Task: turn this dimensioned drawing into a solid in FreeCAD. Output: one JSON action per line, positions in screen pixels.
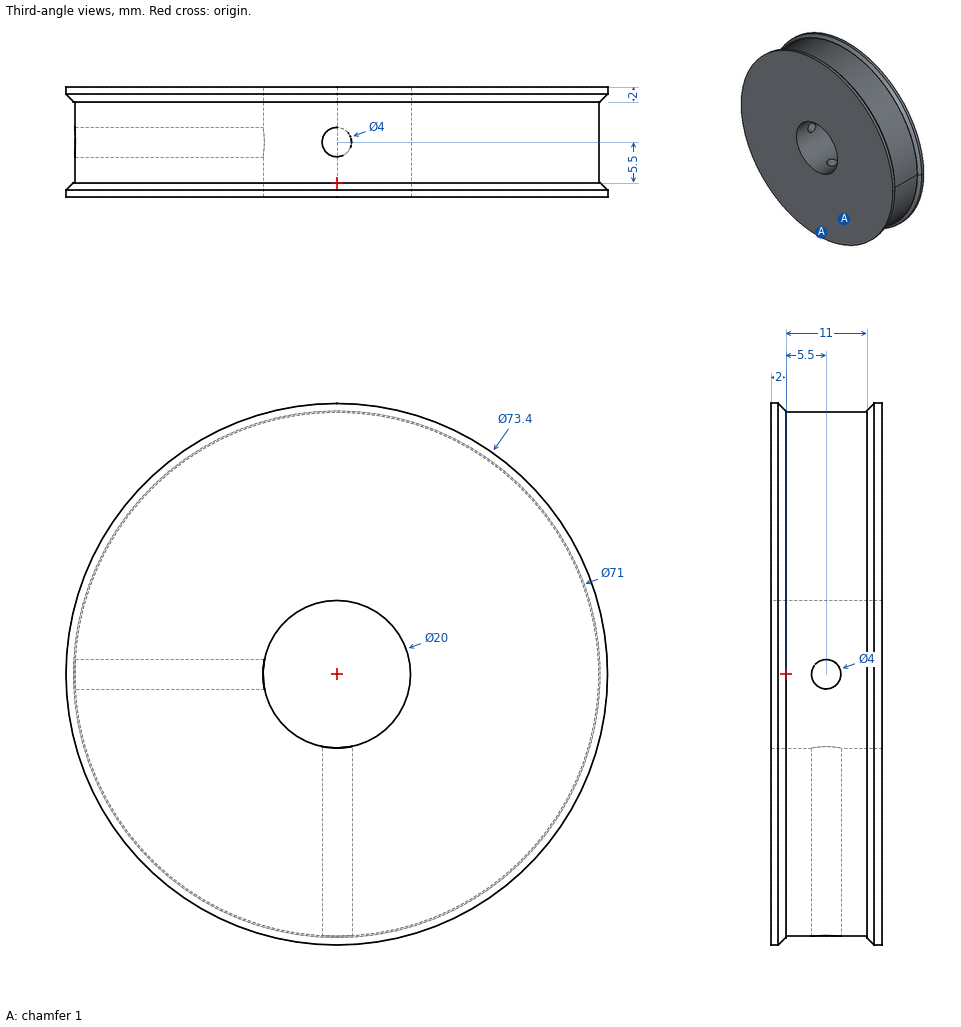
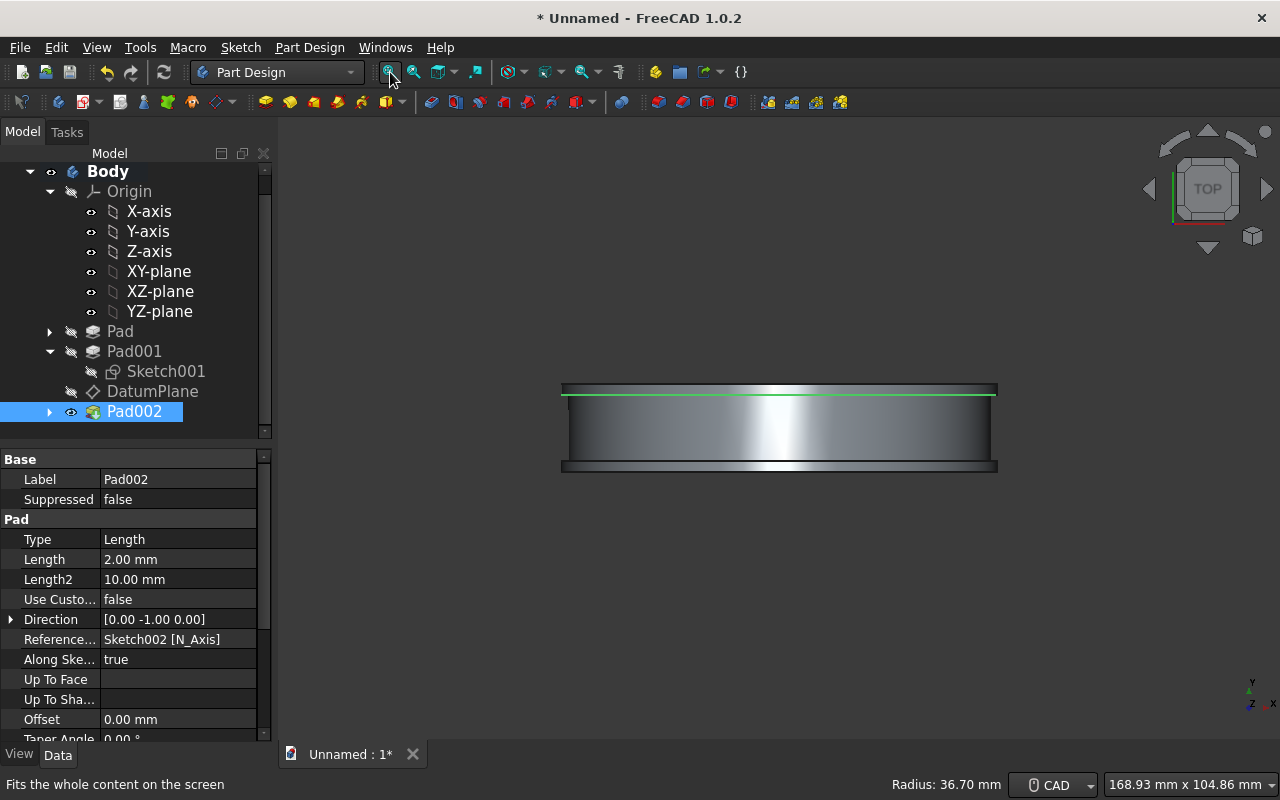
{"action": "left_click", "coordinate": [603, 460], "text": "ctrl"}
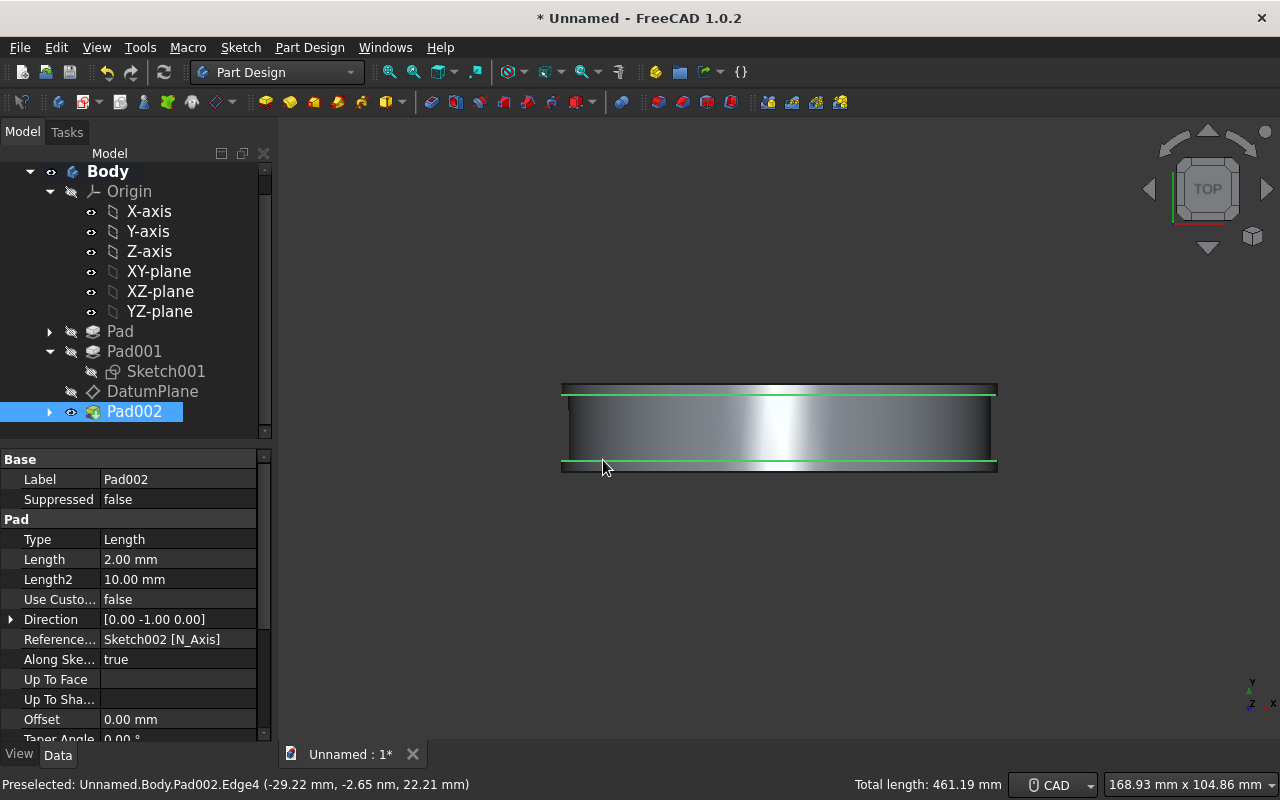
{"action": "left_click", "coordinate": [684, 102]}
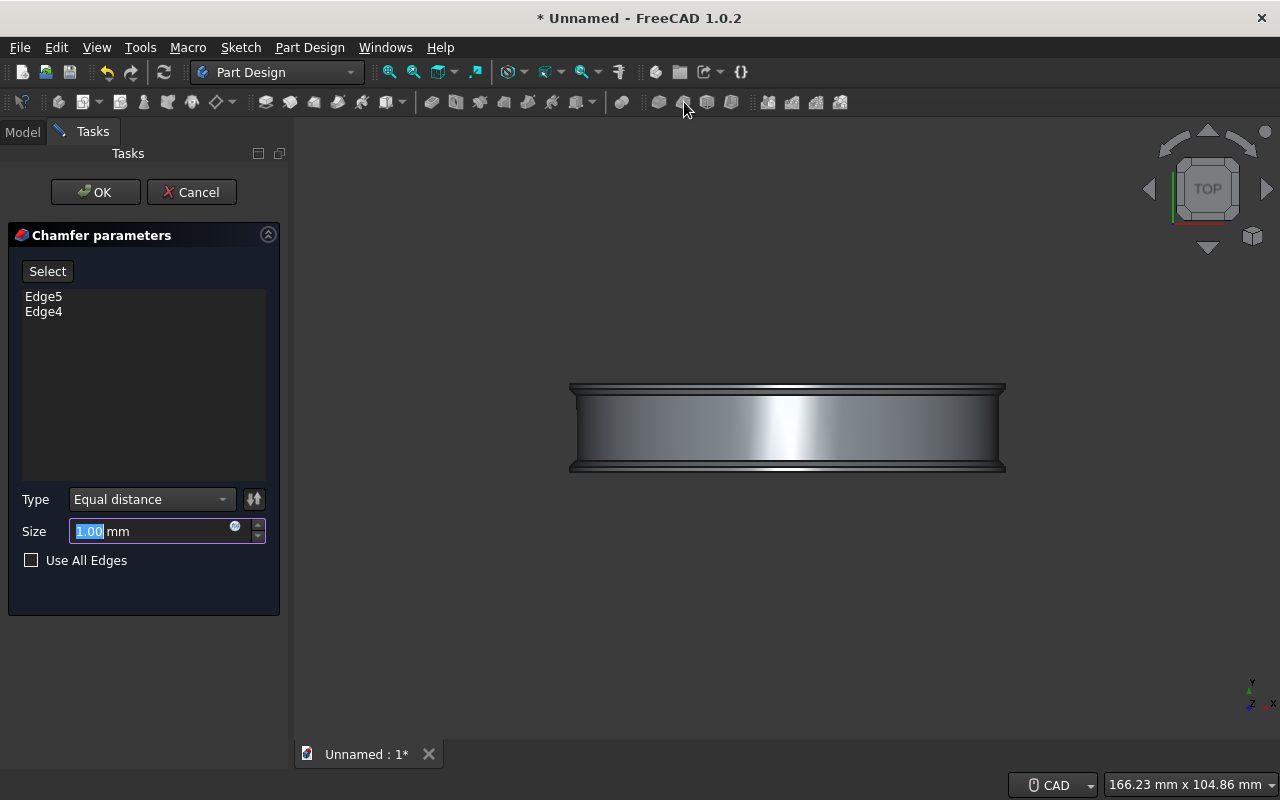
{"action": "type", "text": "1"}
{"action": "key", "text": "Tab"}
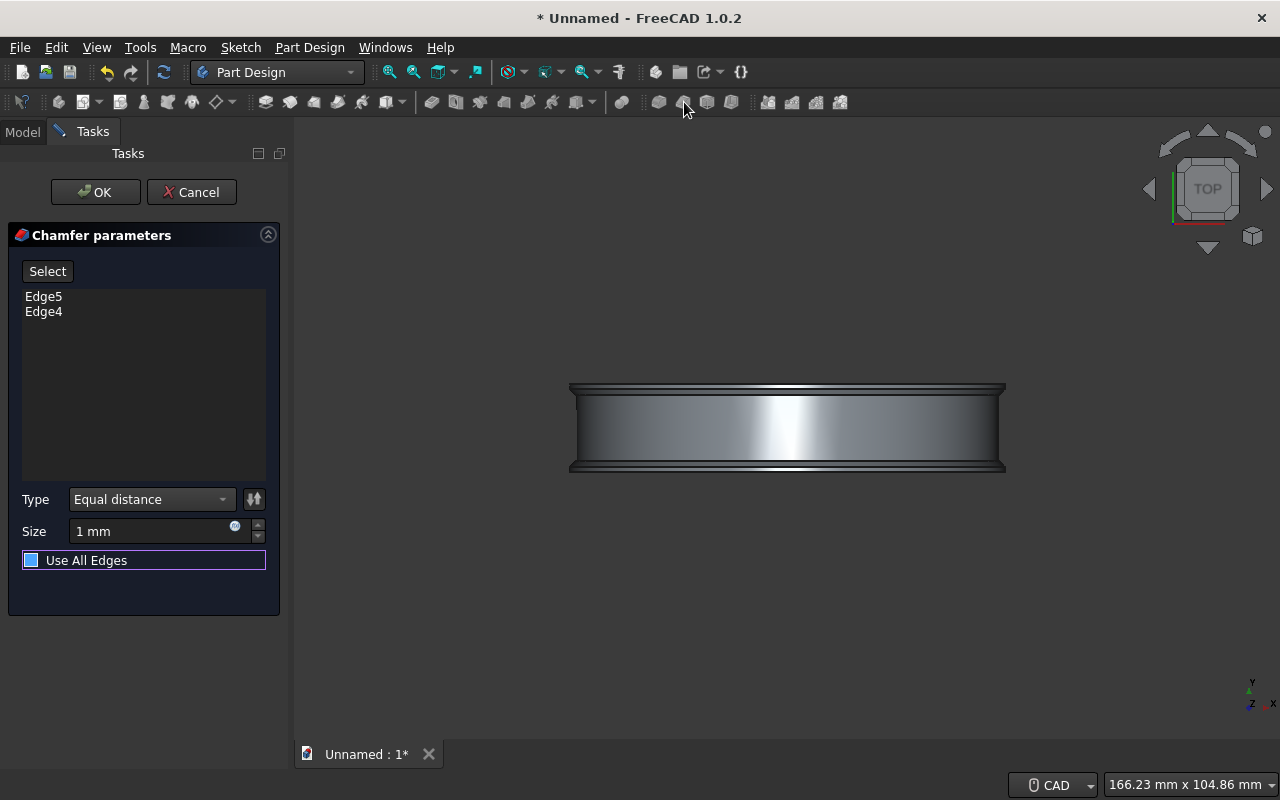
{"action": "left_click", "coordinate": [96, 192]}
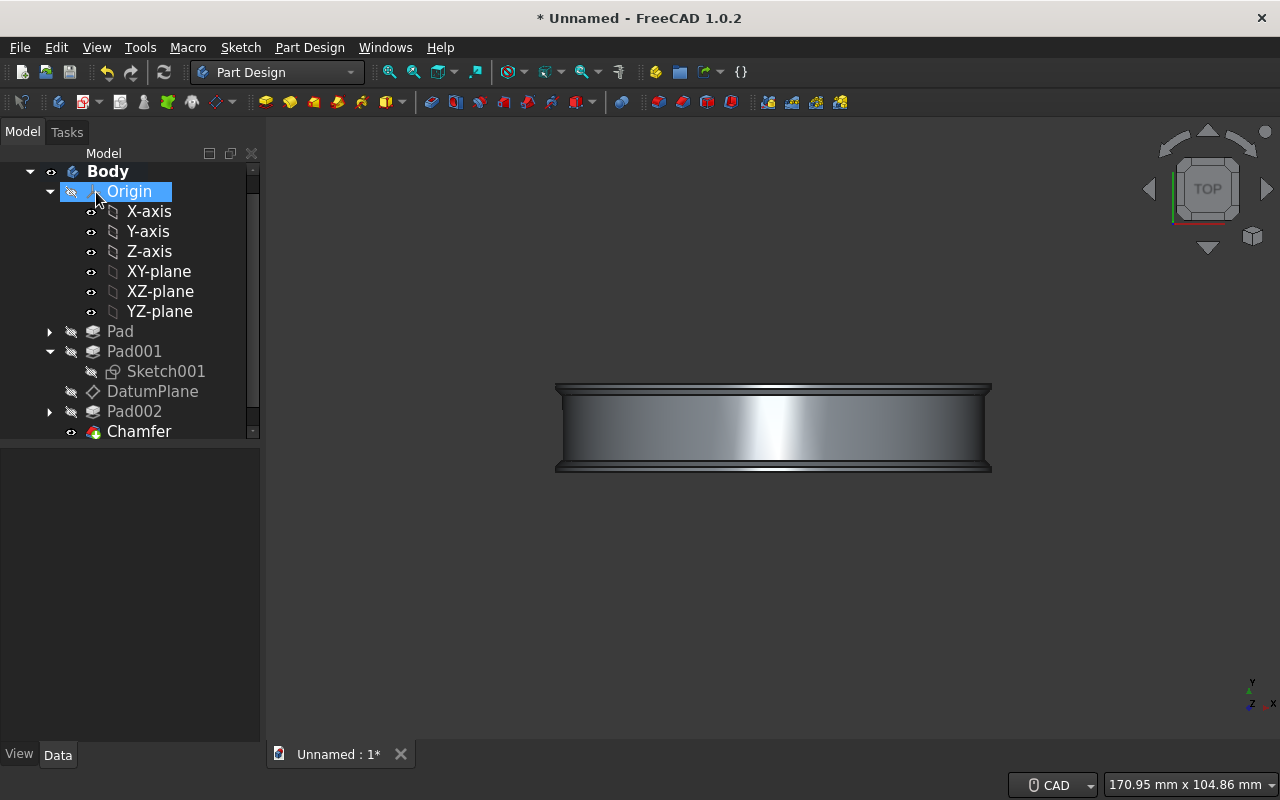
{"action": "left_click", "coordinate": [390, 72]}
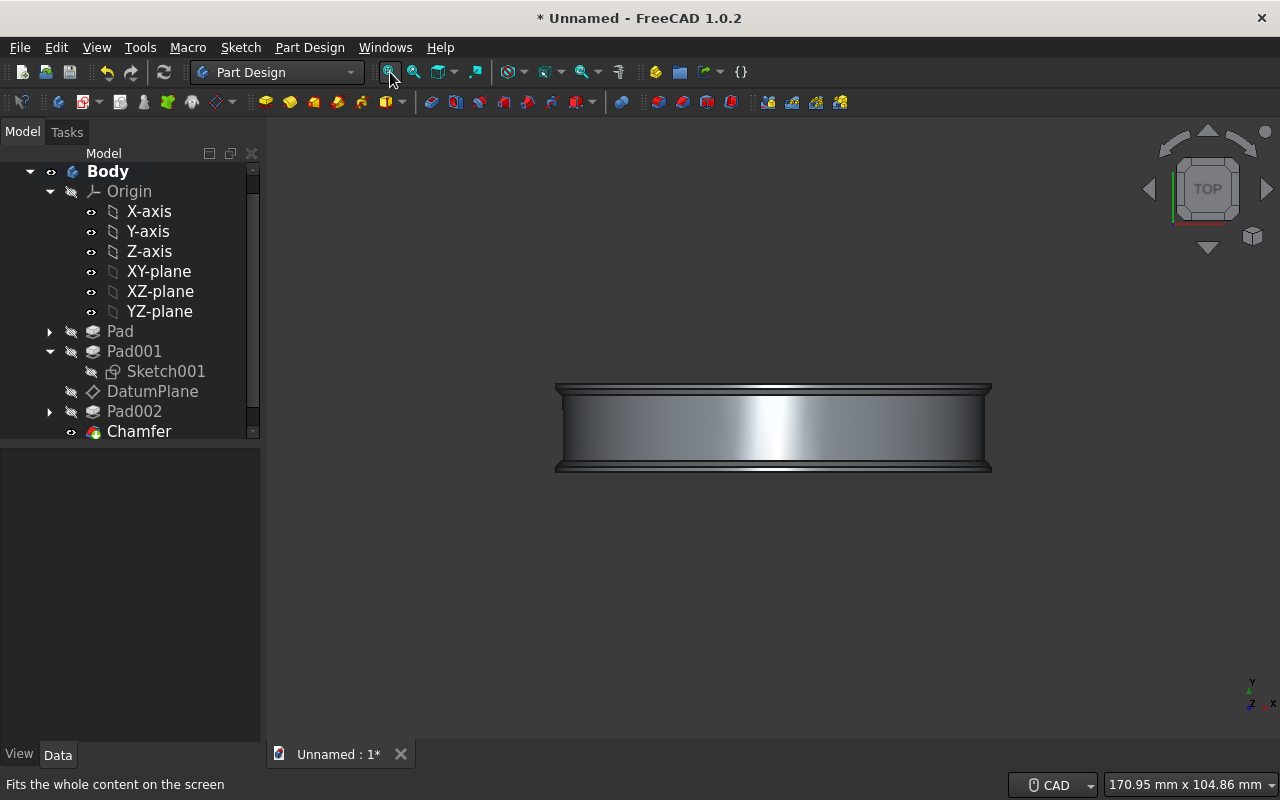
{"action": "left_click", "coordinate": [84, 102]}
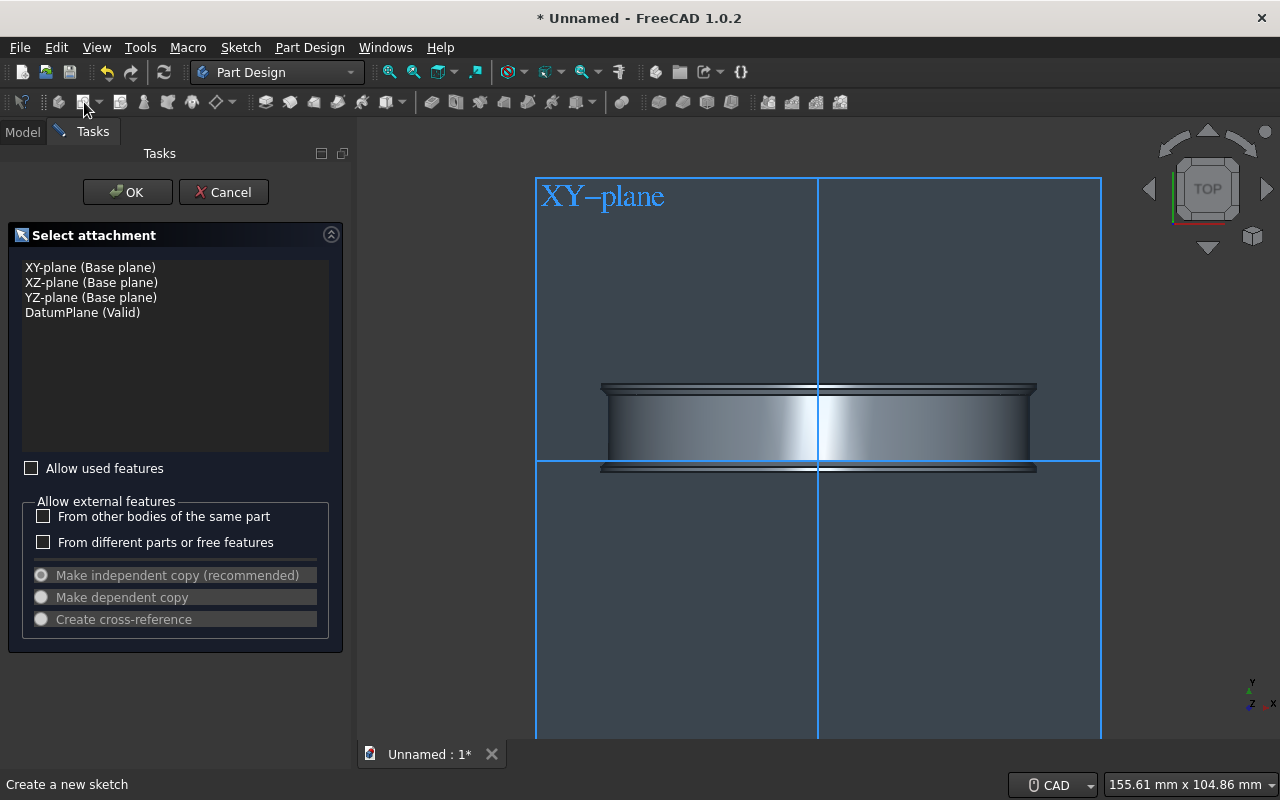
{"action": "left_click", "coordinate": [82, 268]}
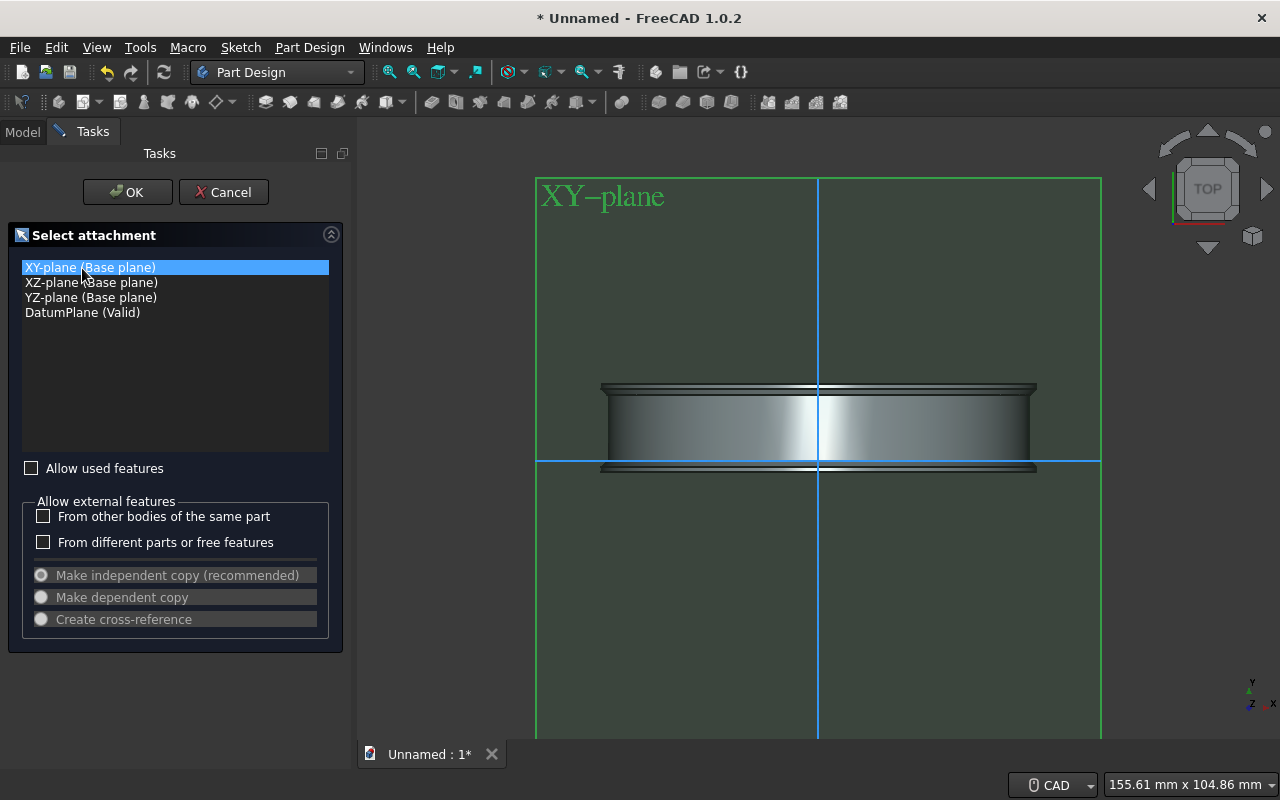
{"action": "left_click", "coordinate": [128, 192]}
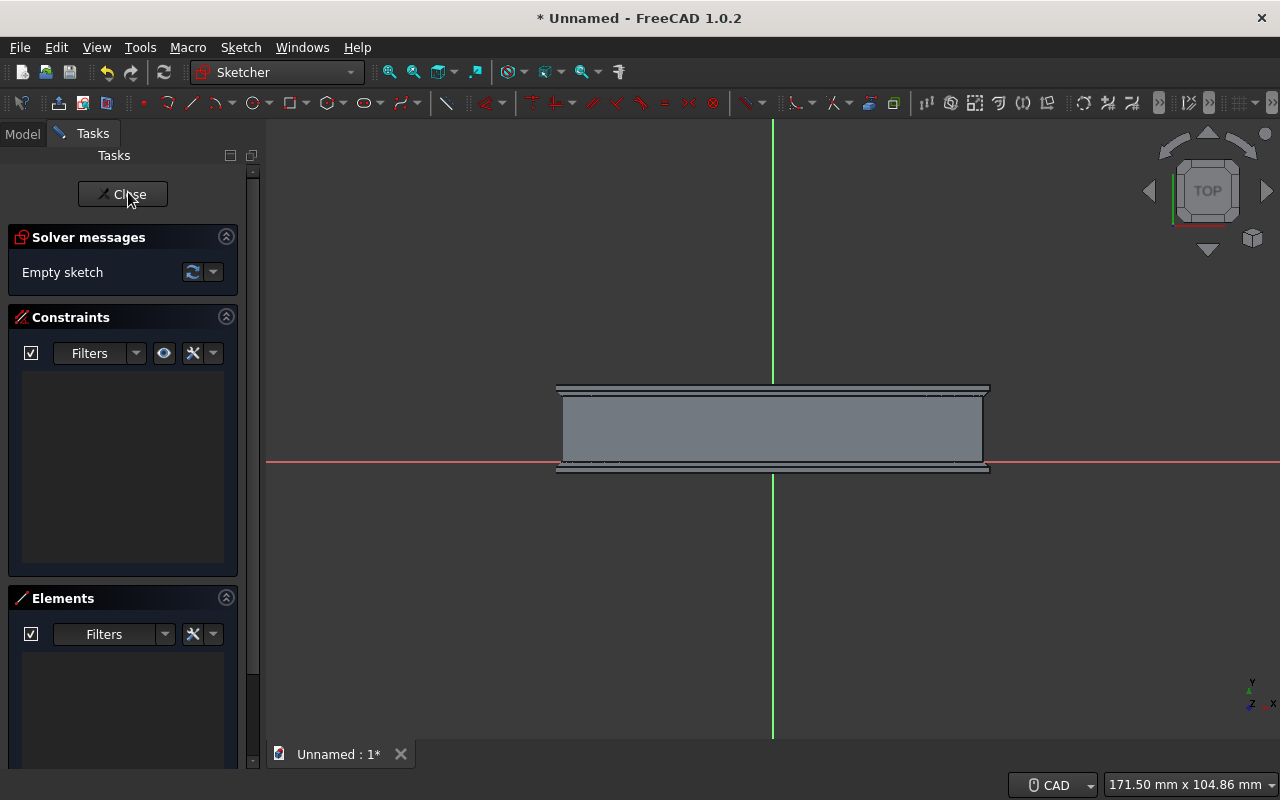
{"action": "left_click", "coordinate": [108, 104]}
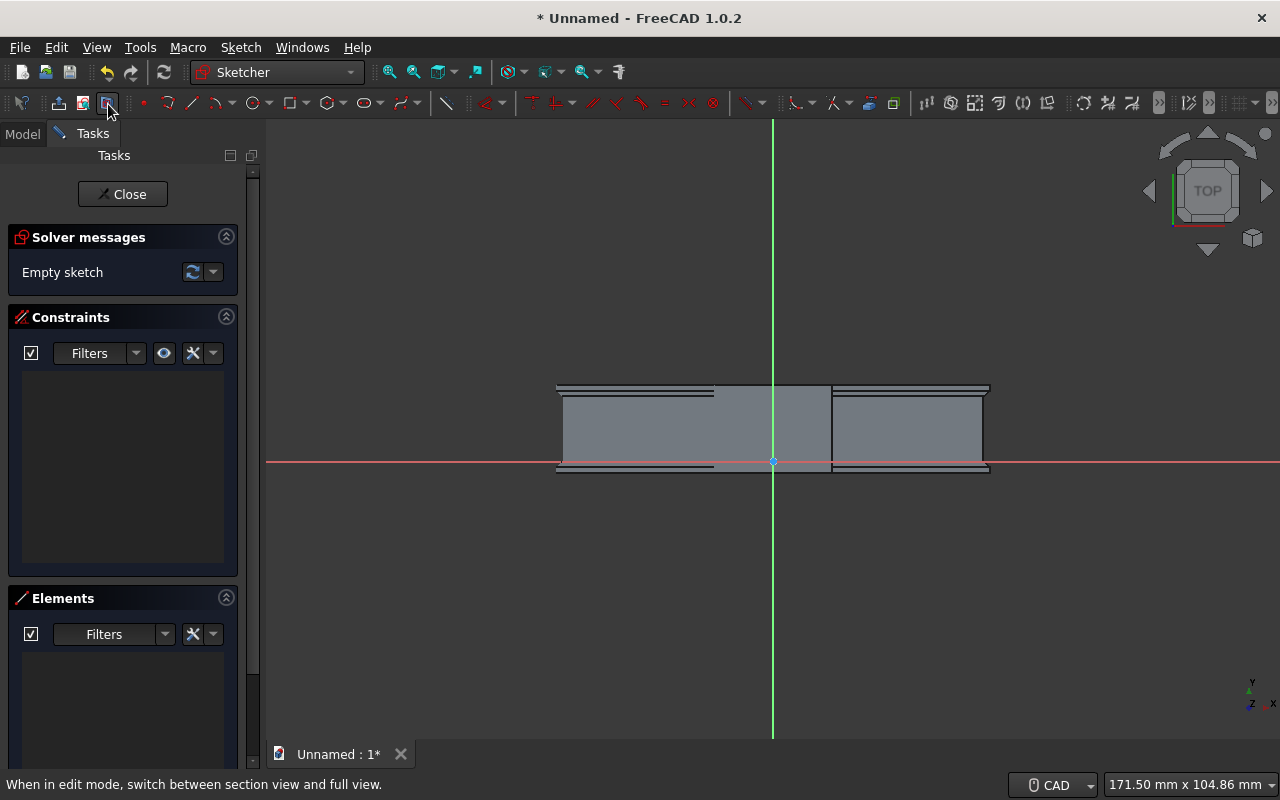
{"action": "scroll", "coordinate": [782, 441], "scroll_direction": "up", "scroll_amount": 11}